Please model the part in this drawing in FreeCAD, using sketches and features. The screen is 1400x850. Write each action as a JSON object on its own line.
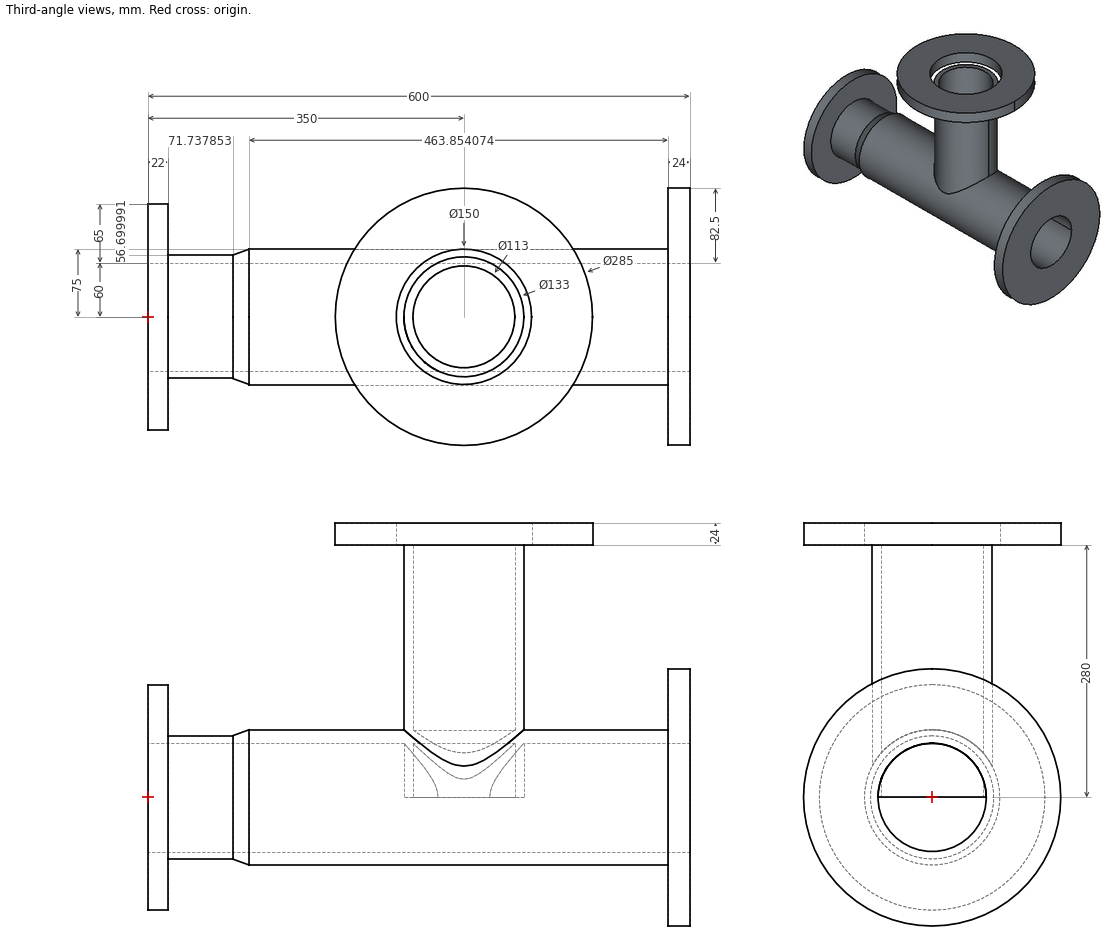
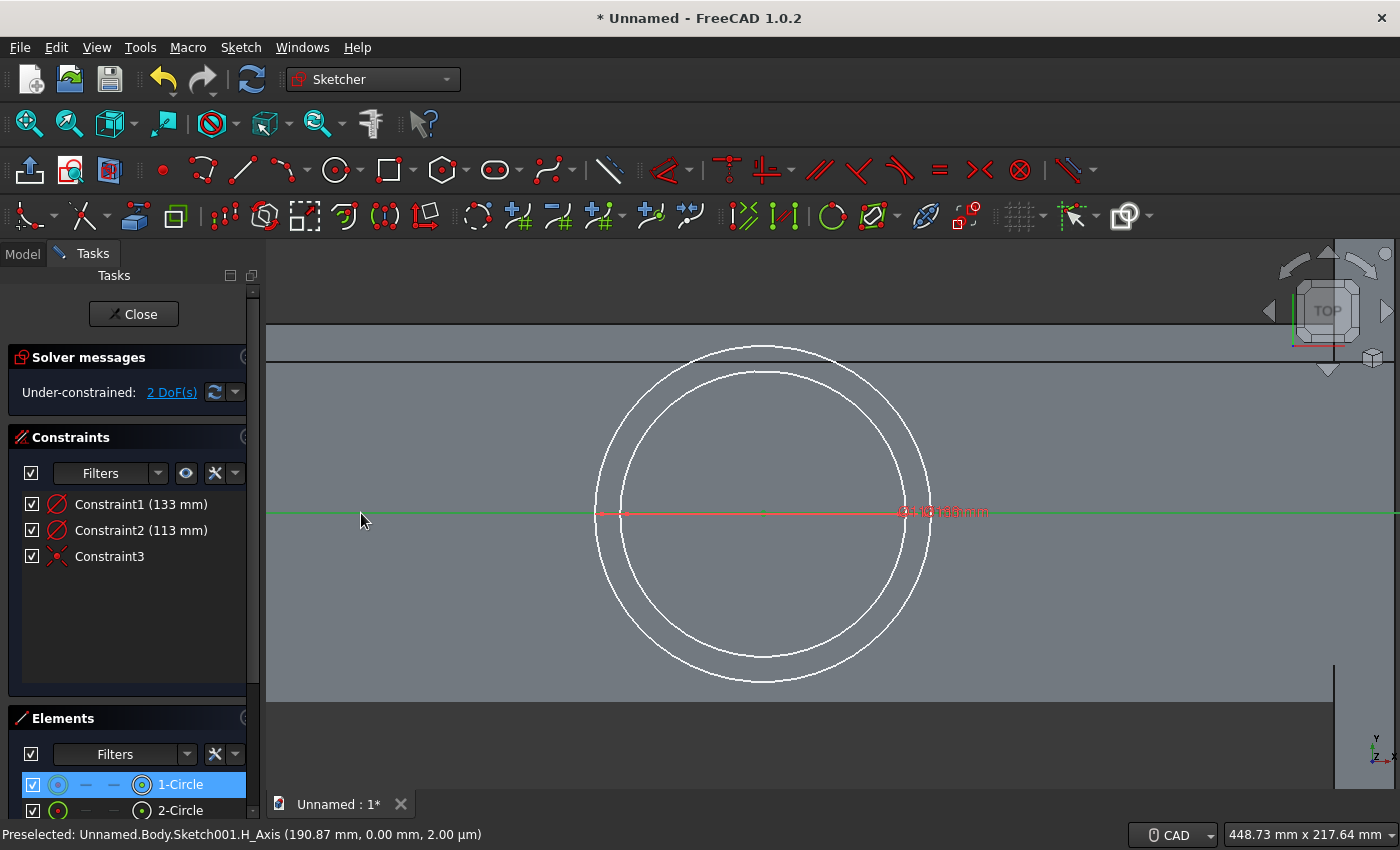
{"action": "key", "text": "c"}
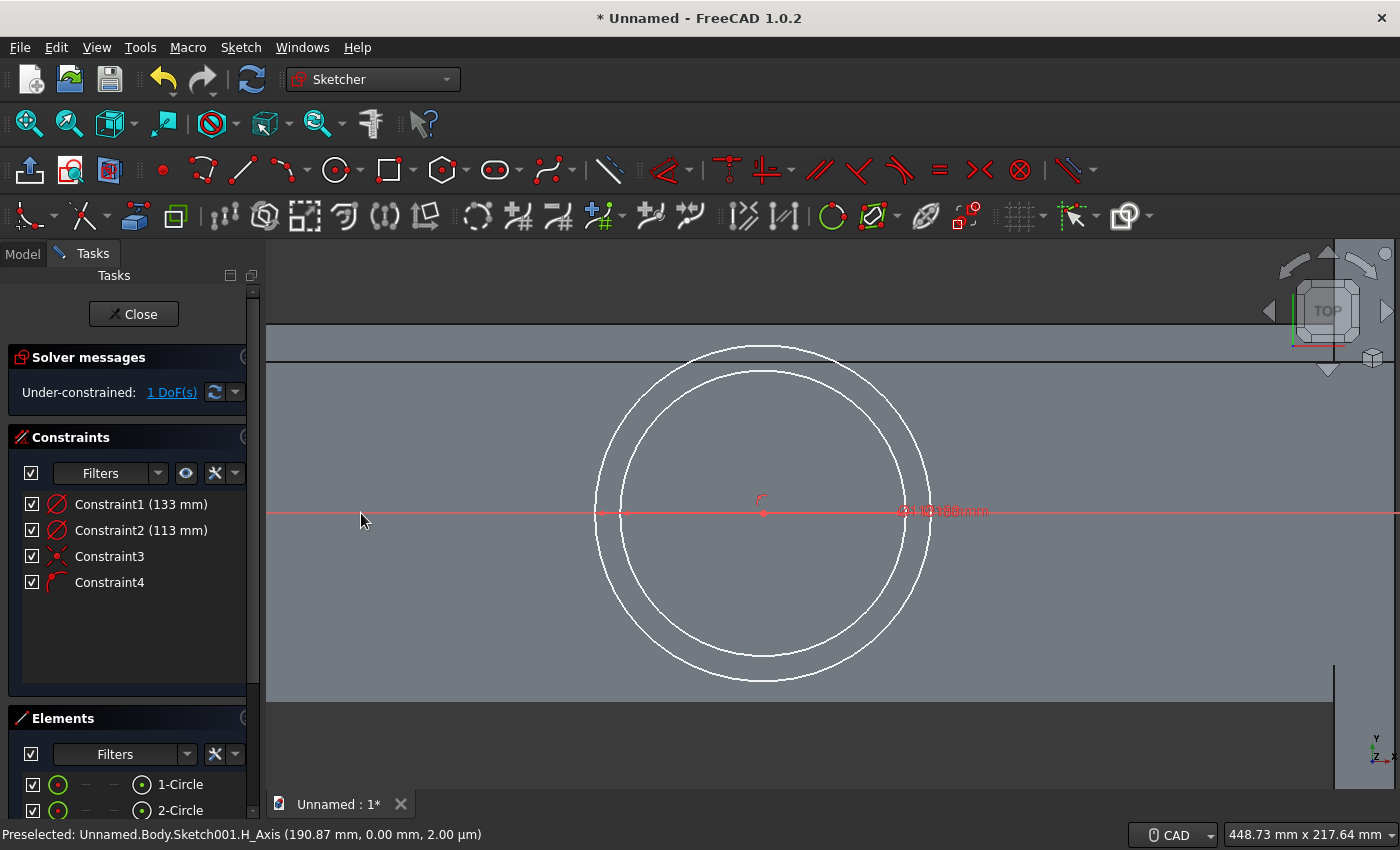
{"action": "key", "text": "d"}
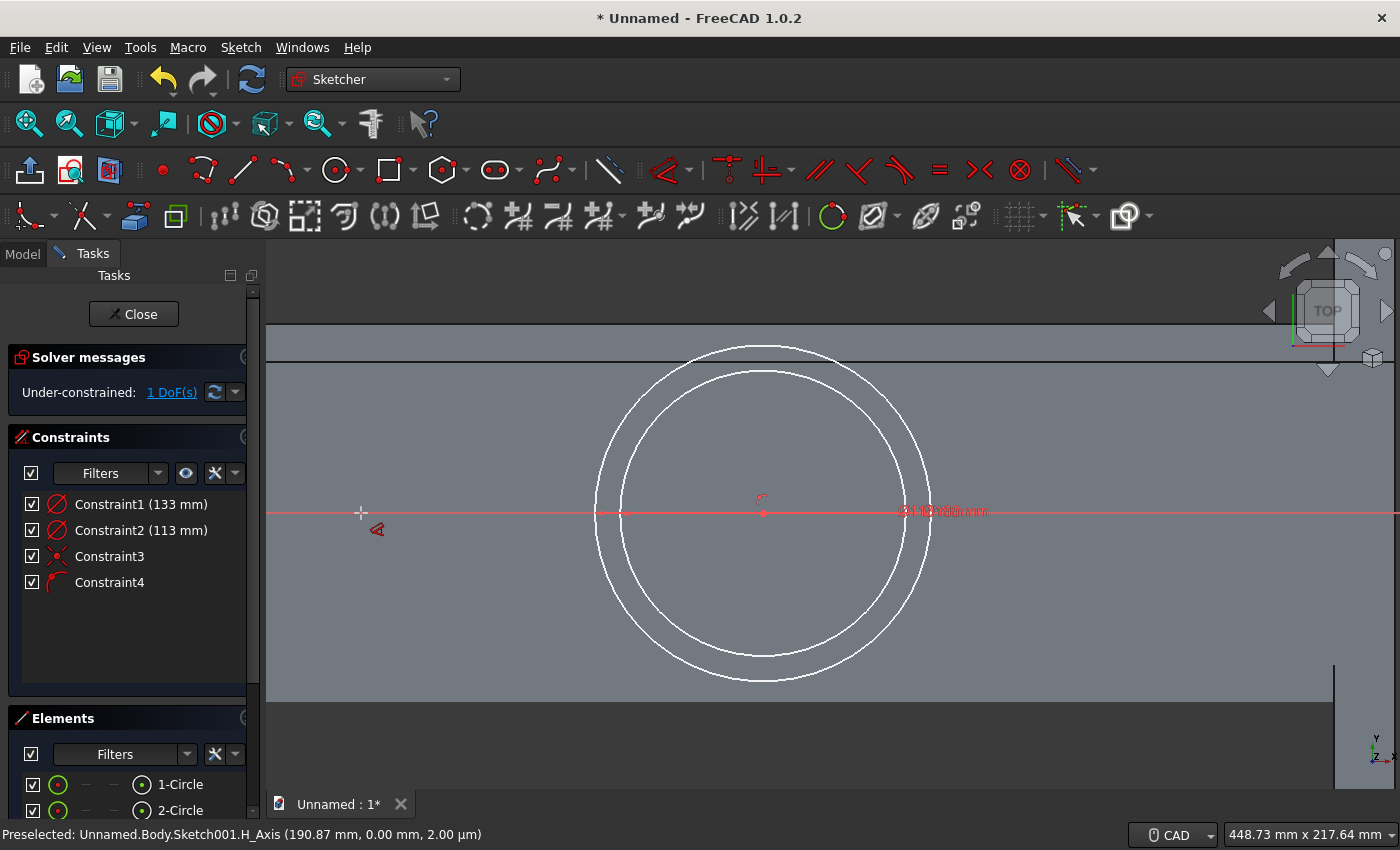
{"action": "left_click", "coordinate": [763, 513]}
{"action": "left_click", "coordinate": [528, 547]}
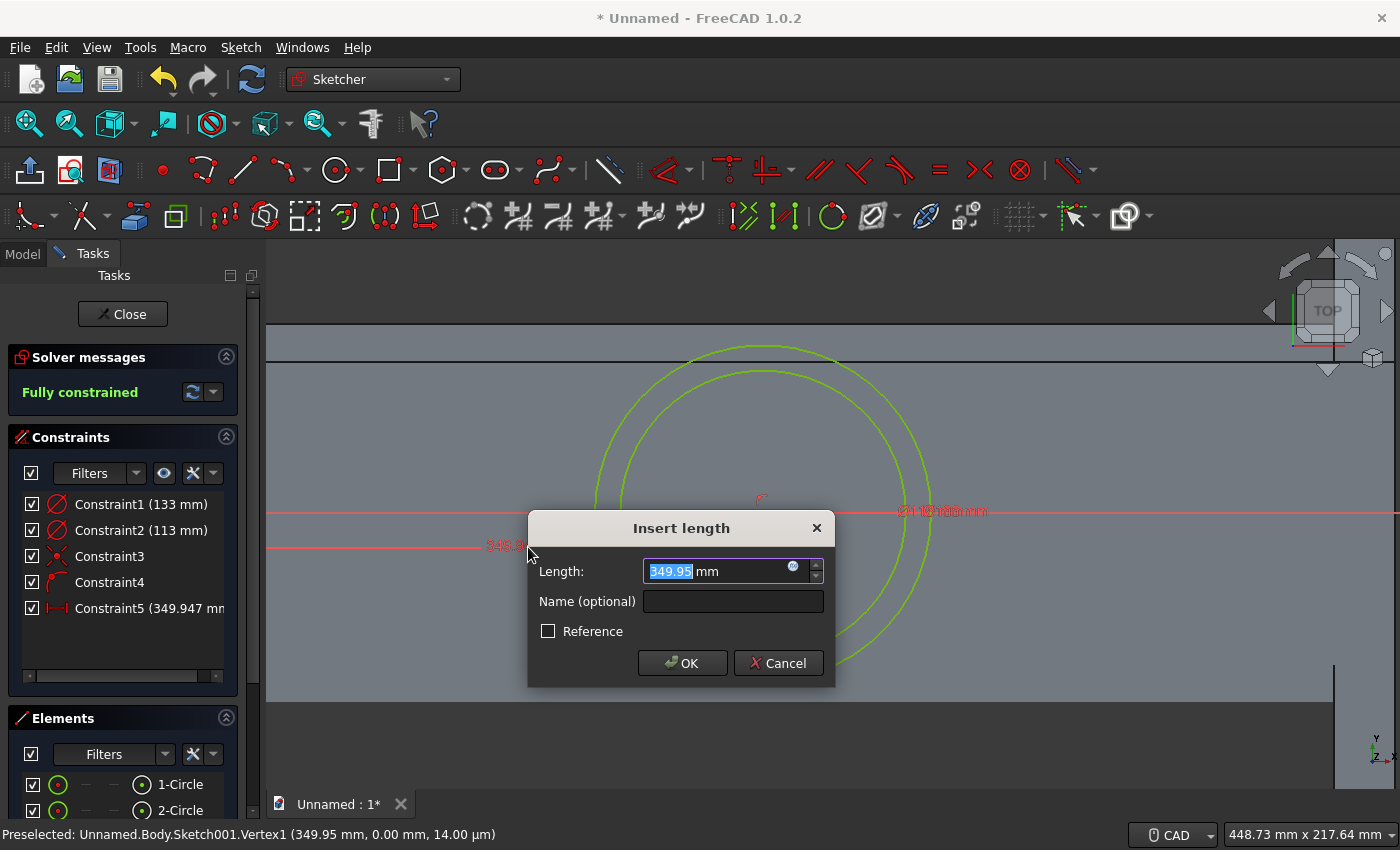
{"action": "type", "text": "350"}
{"action": "key", "text": "Return"}
{"action": "key", "text": "Escape"}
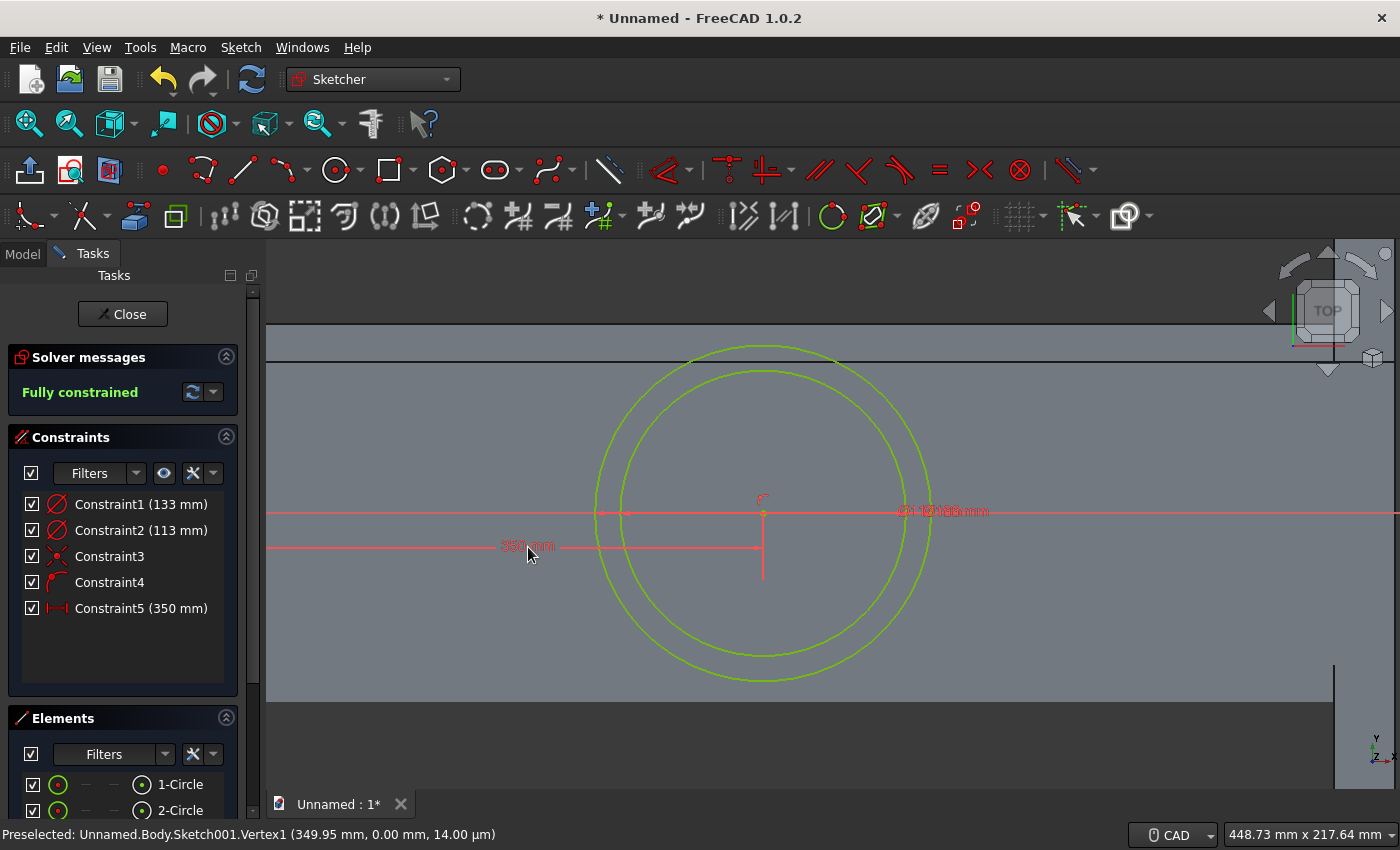
{"action": "left_click", "coordinate": [123, 314]}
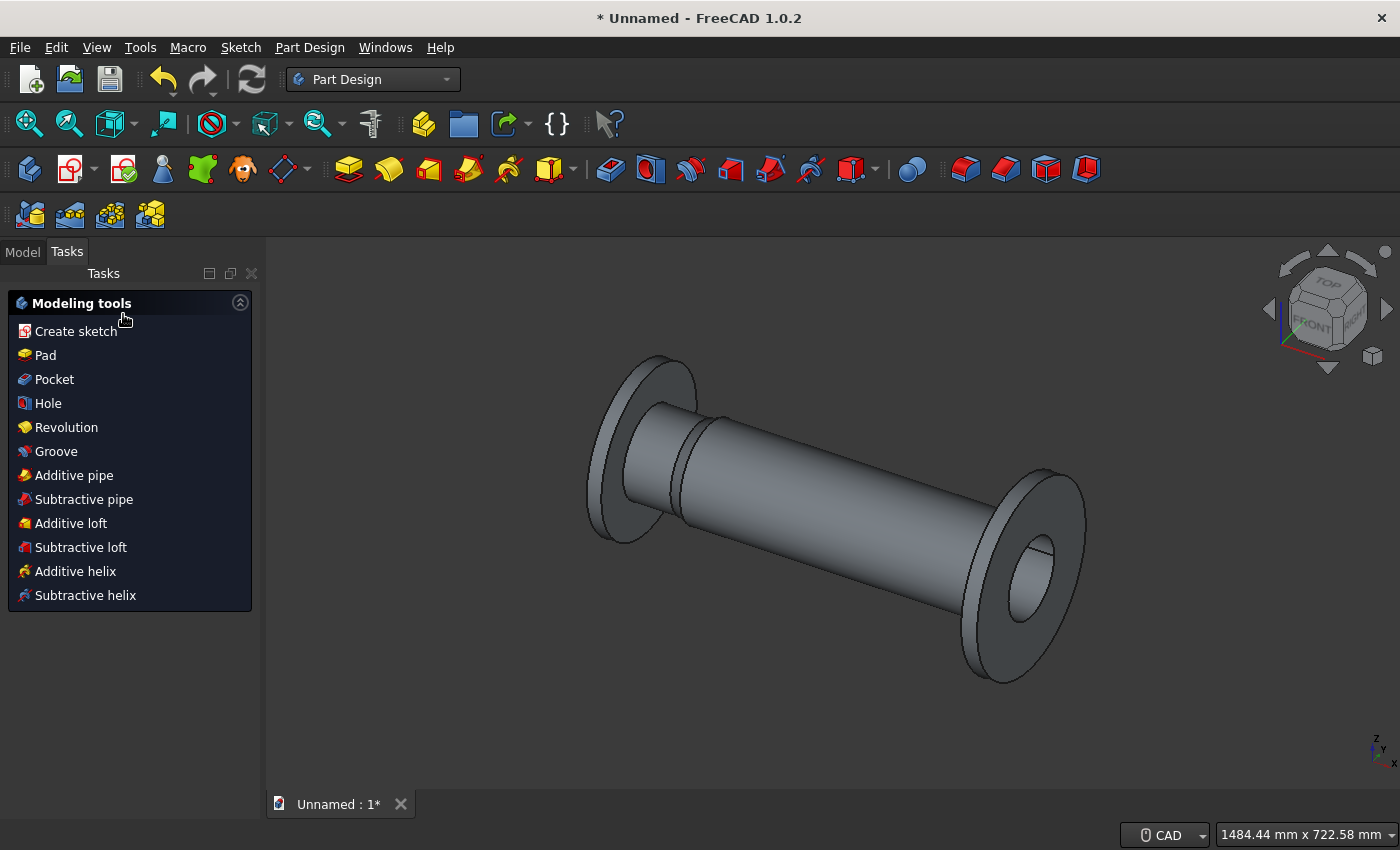
{"action": "left_click", "coordinate": [350, 170]}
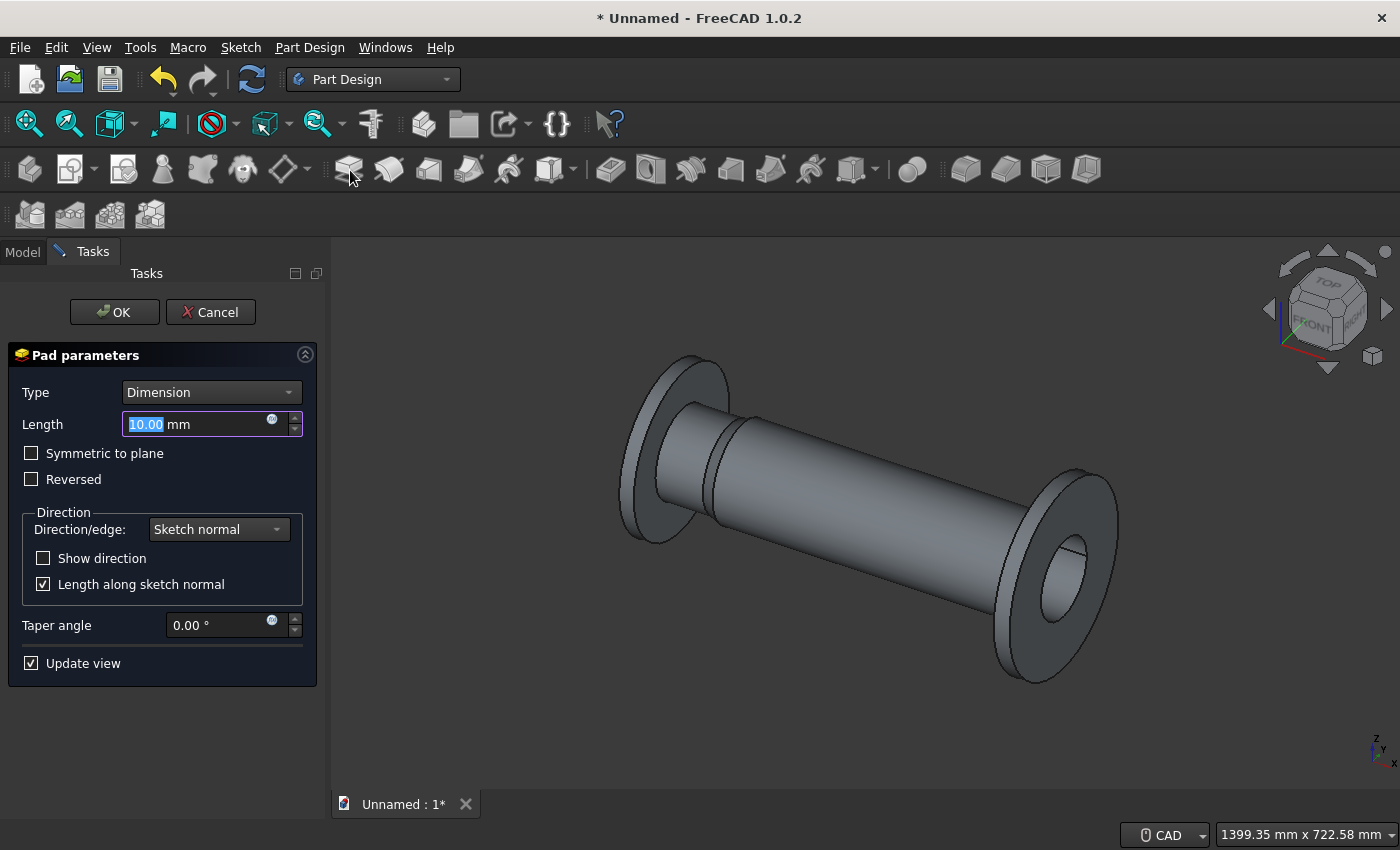
{"action": "type", "text": "280"}
{"action": "key", "text": "Tab"}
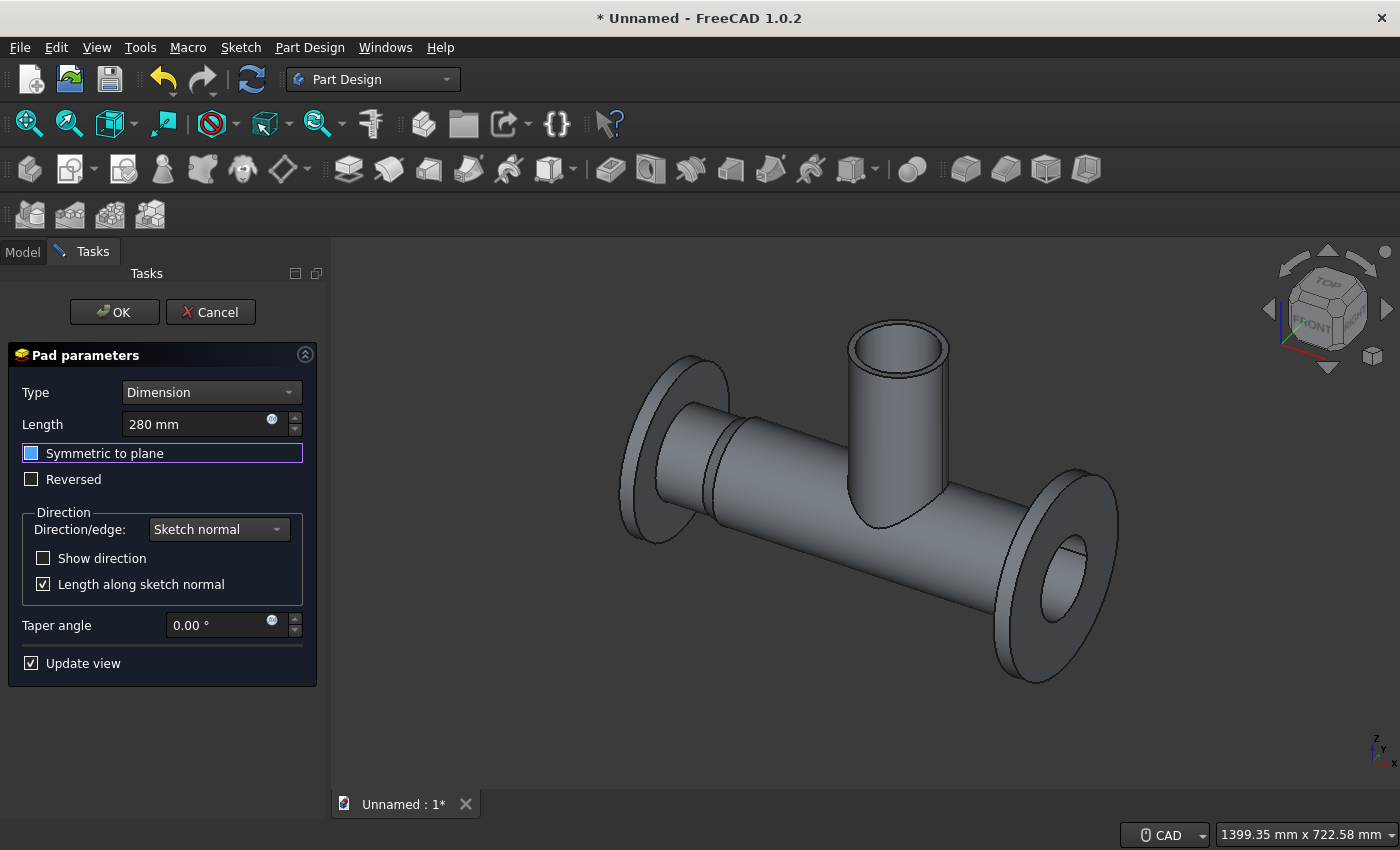
{"action": "left_click", "coordinate": [115, 312]}